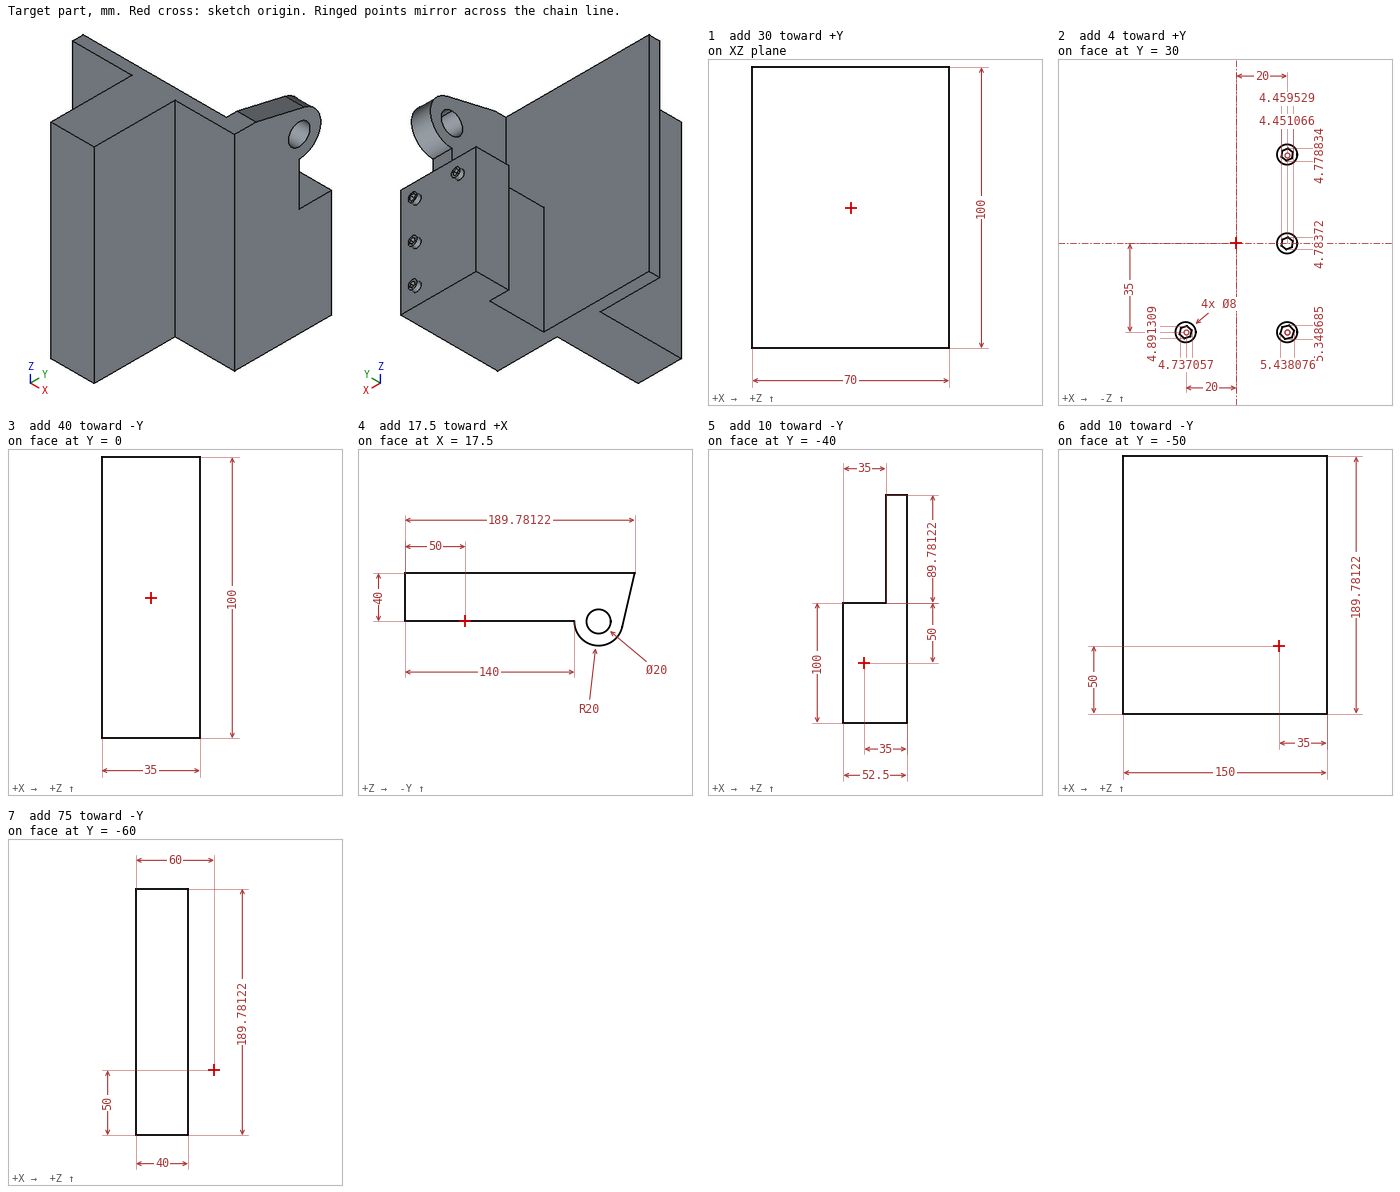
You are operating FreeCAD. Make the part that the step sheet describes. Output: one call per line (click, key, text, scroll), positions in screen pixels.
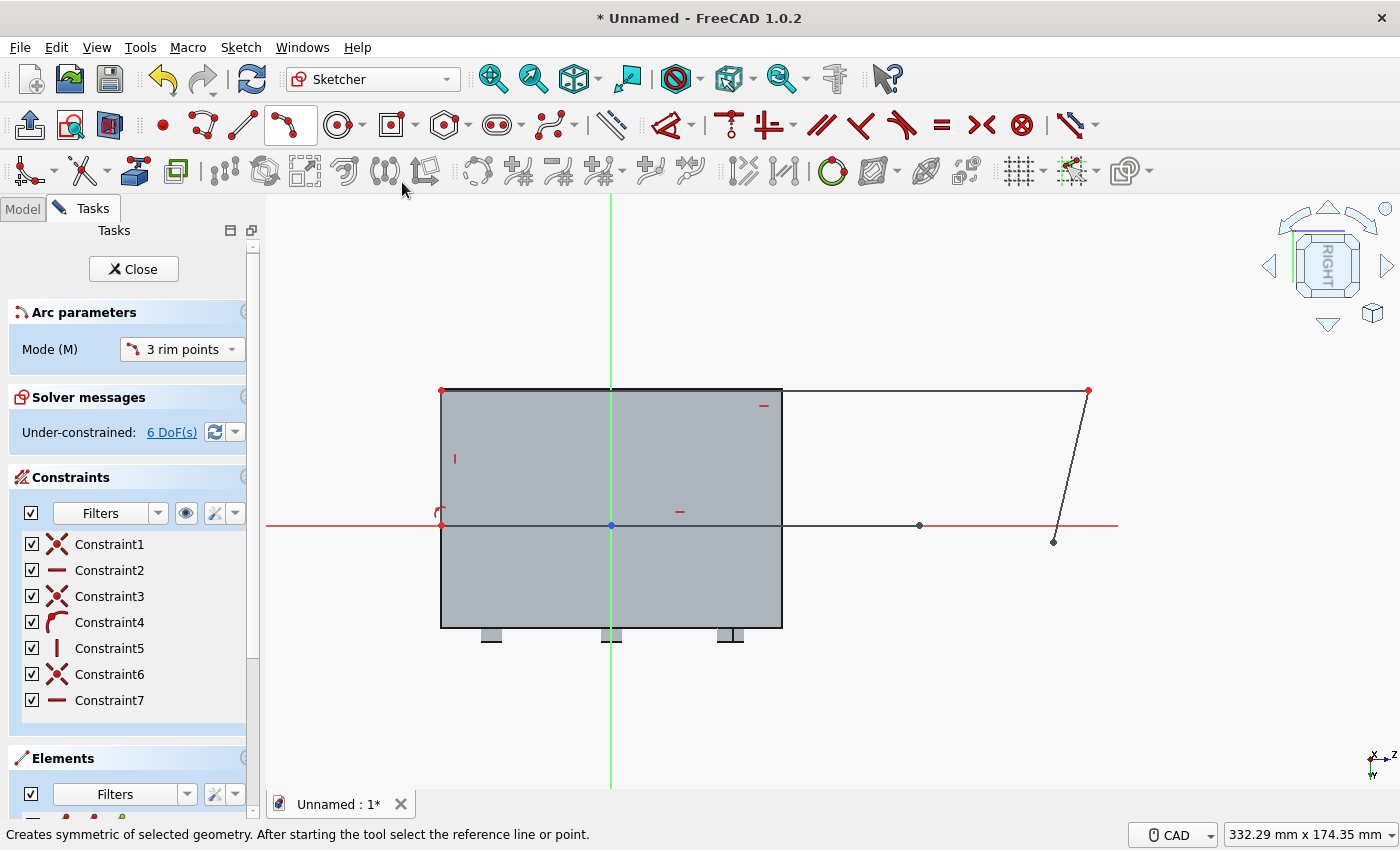
click(919, 526)
click(1053, 542)
click(979, 594)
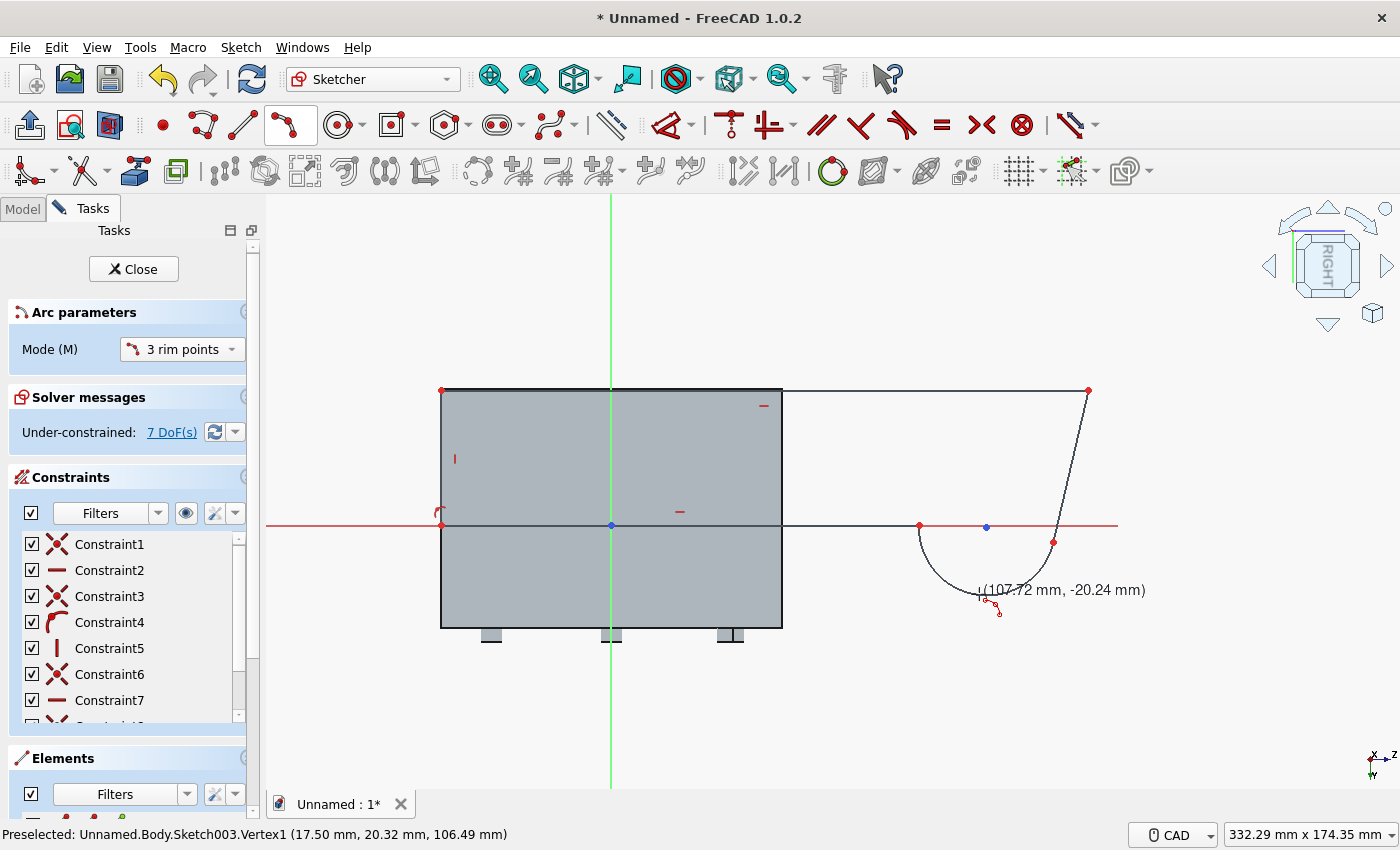
key(g)
key(c)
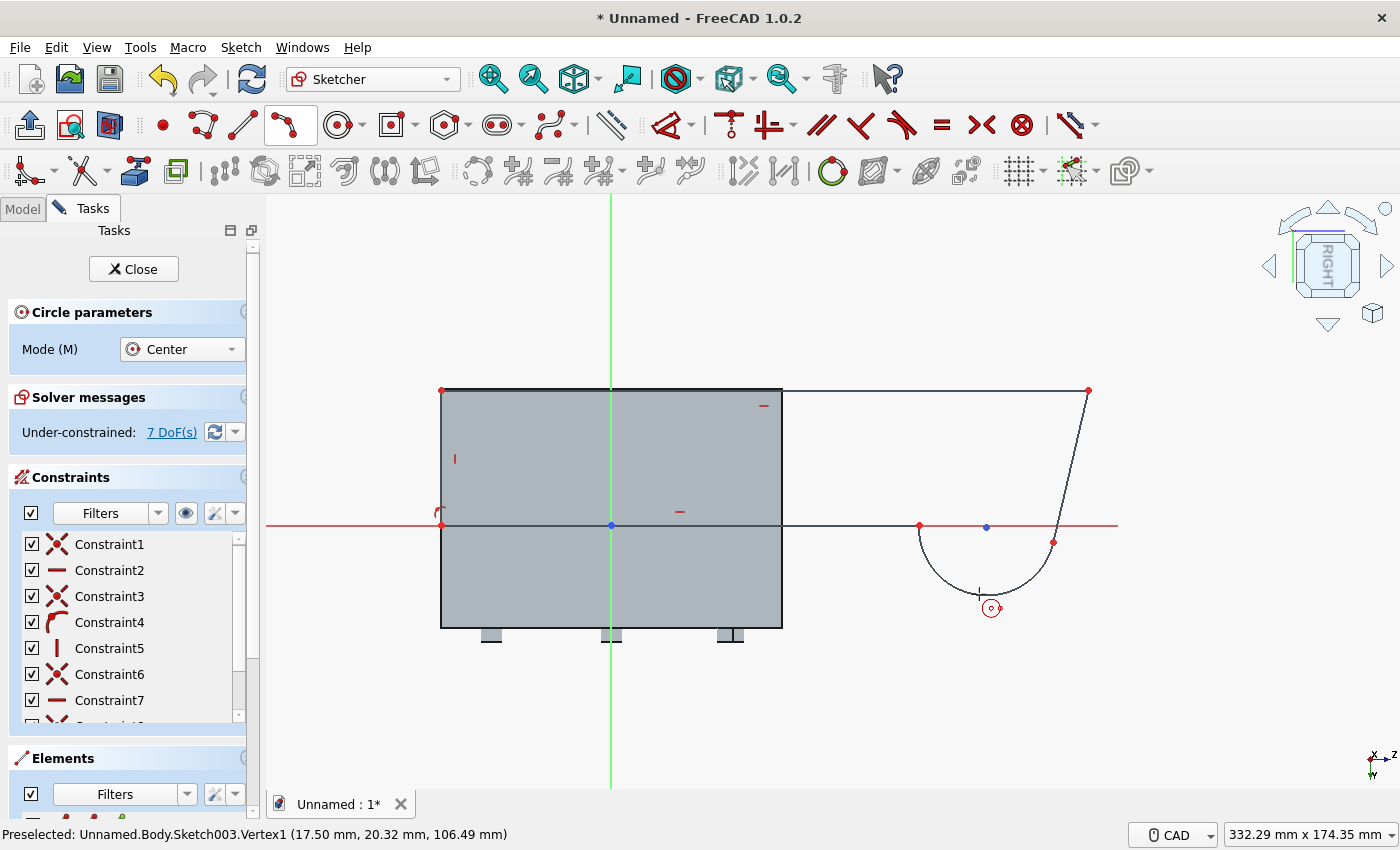
click(987, 526)
move(1011, 502)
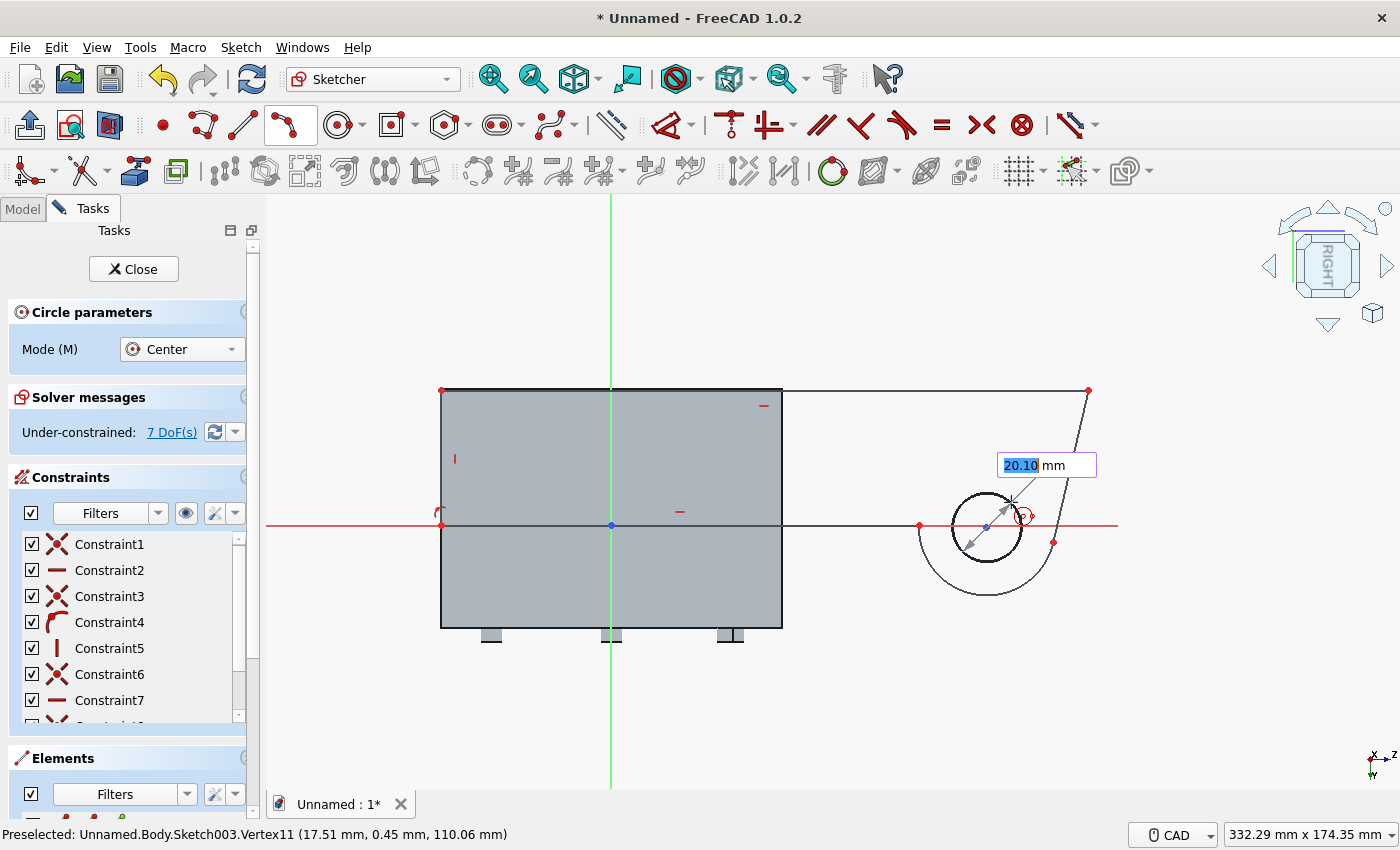
text(20)
key(Return)
key(Escape)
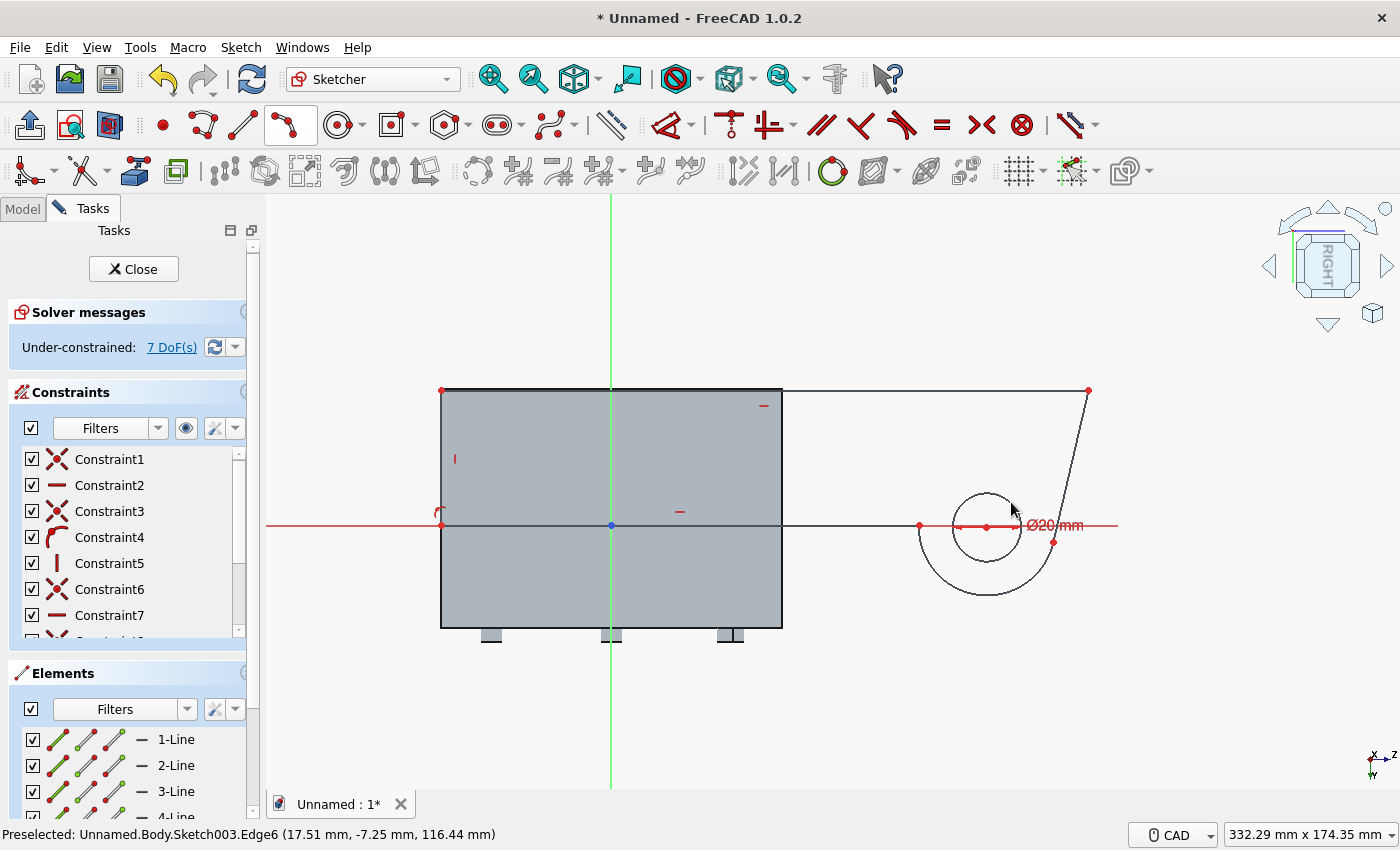
click(1064, 497)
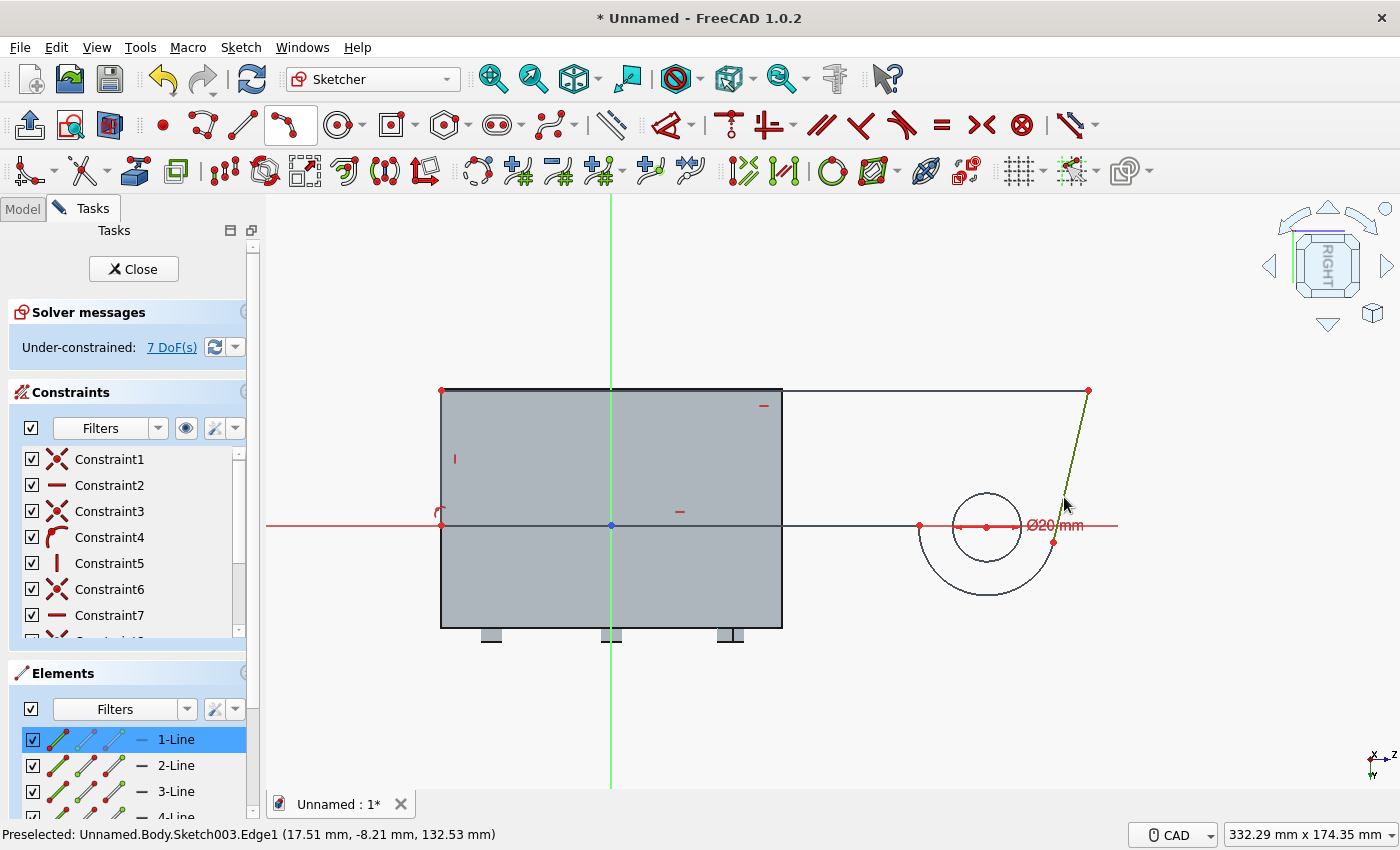
click(943, 579)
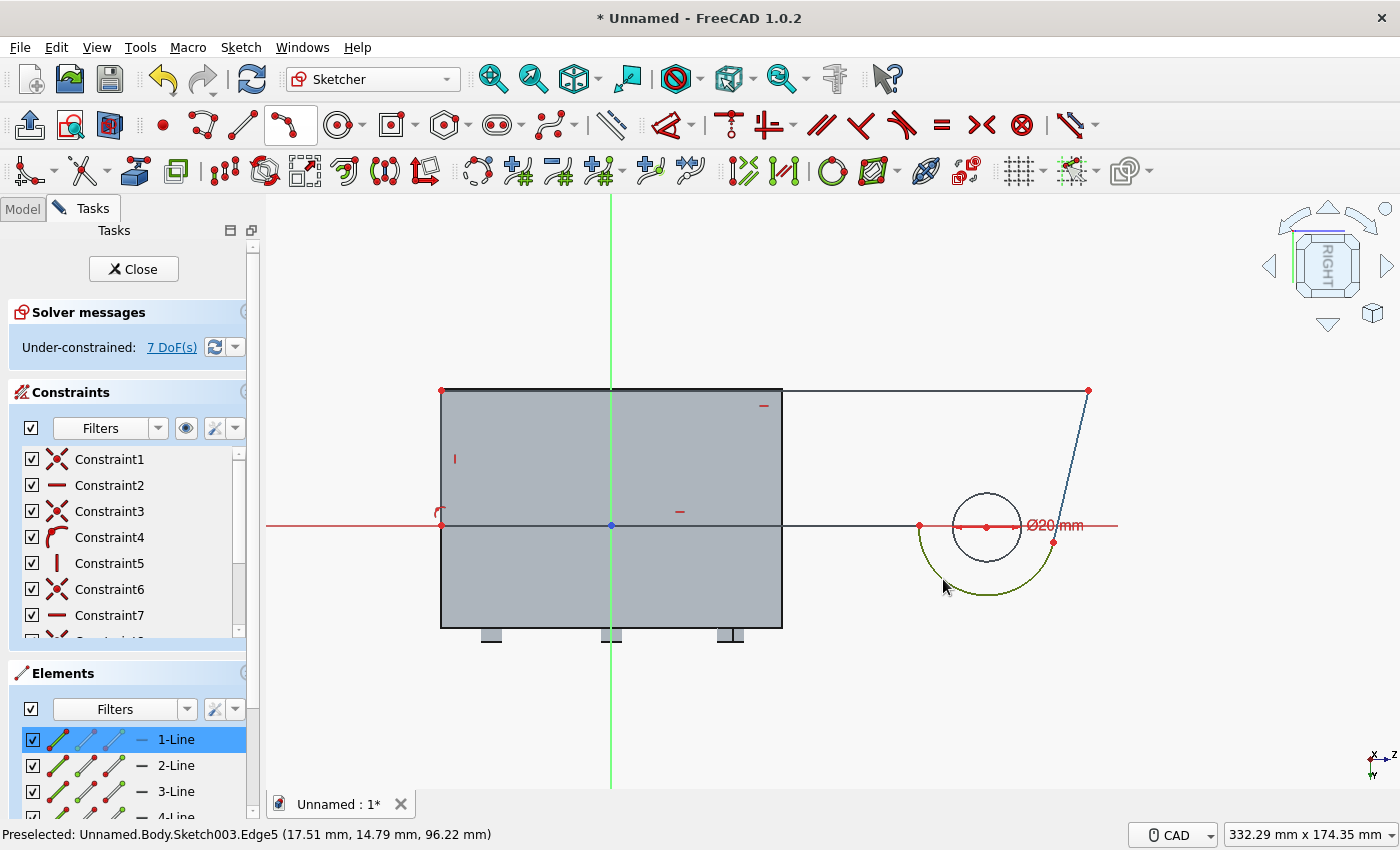
click(902, 126)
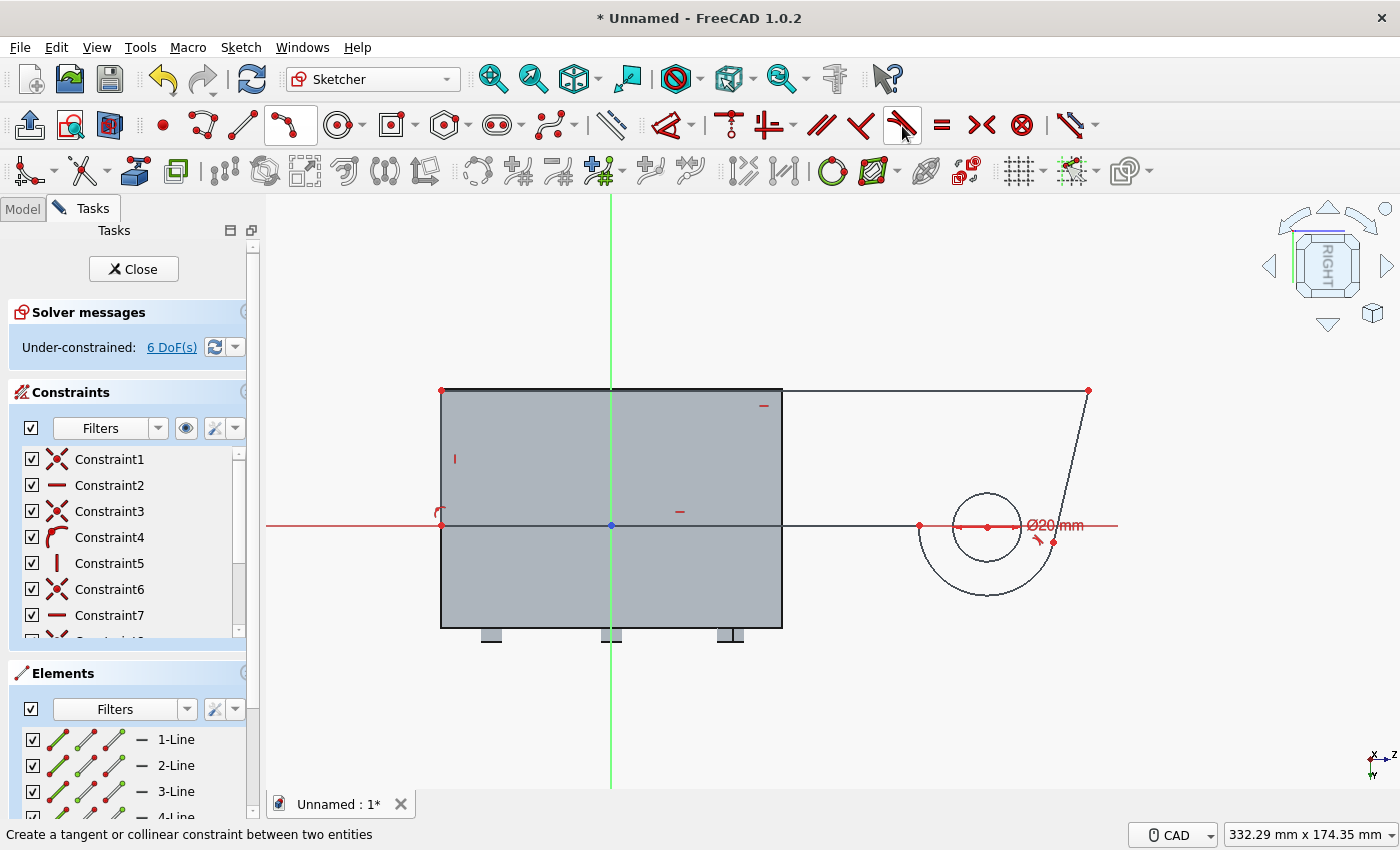
click(987, 527)